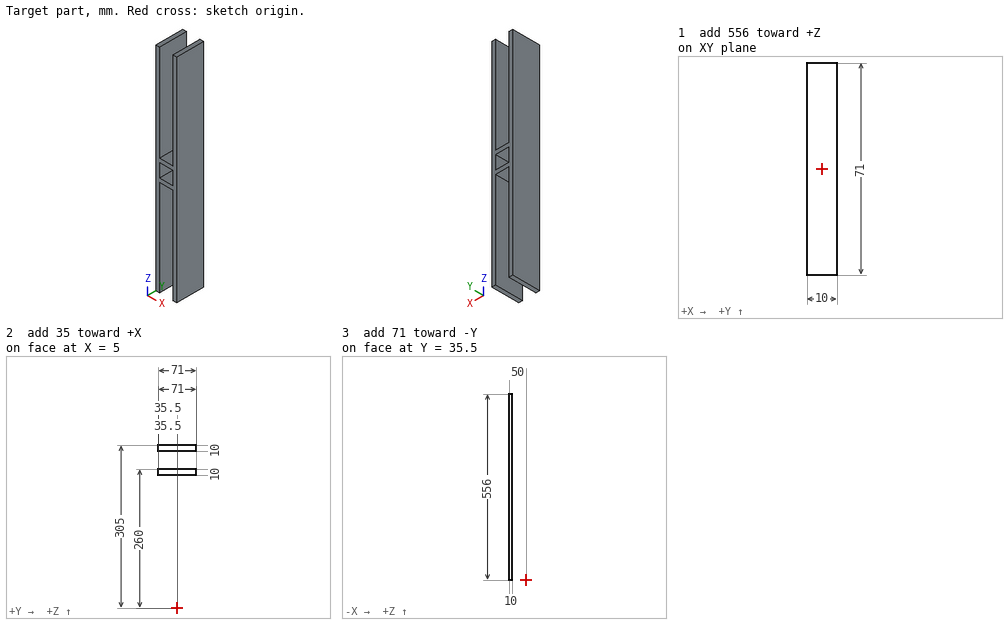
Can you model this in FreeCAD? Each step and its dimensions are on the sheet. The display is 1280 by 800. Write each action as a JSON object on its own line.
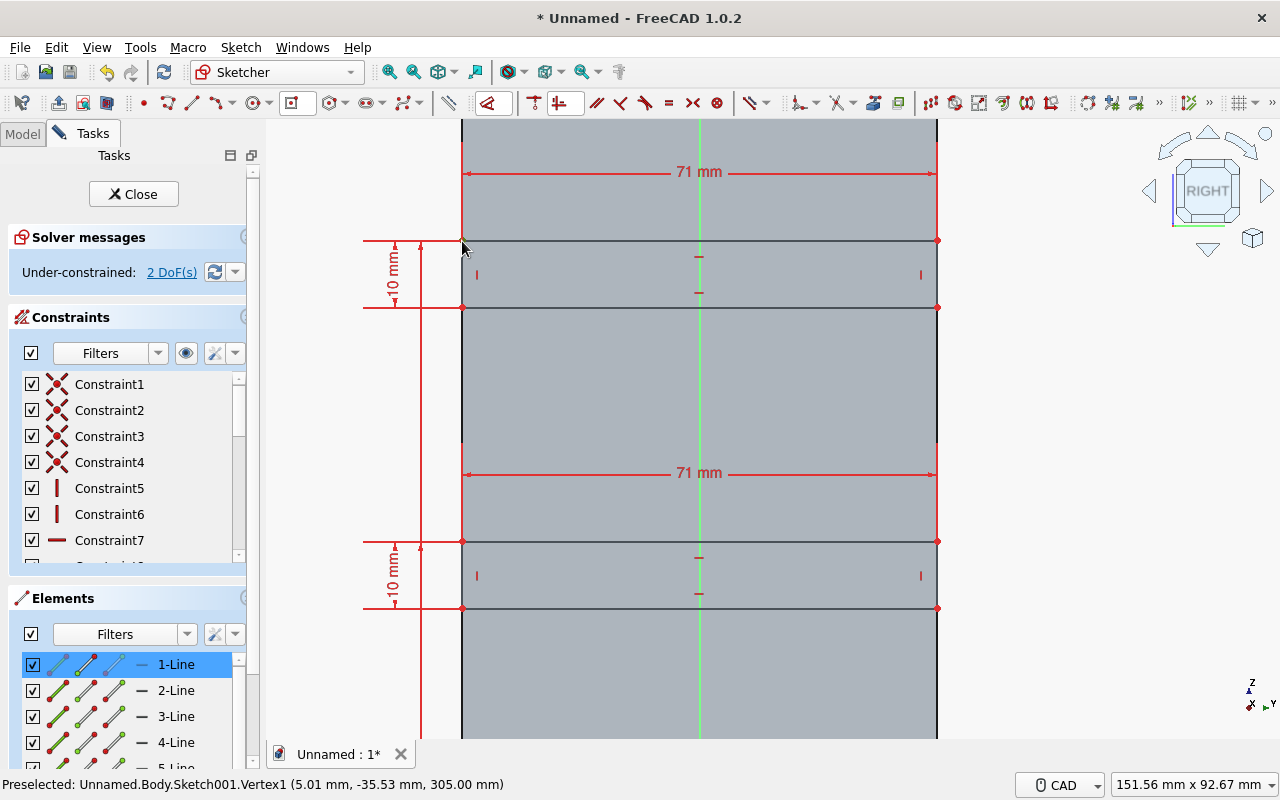
{"action": "key", "text": "l"}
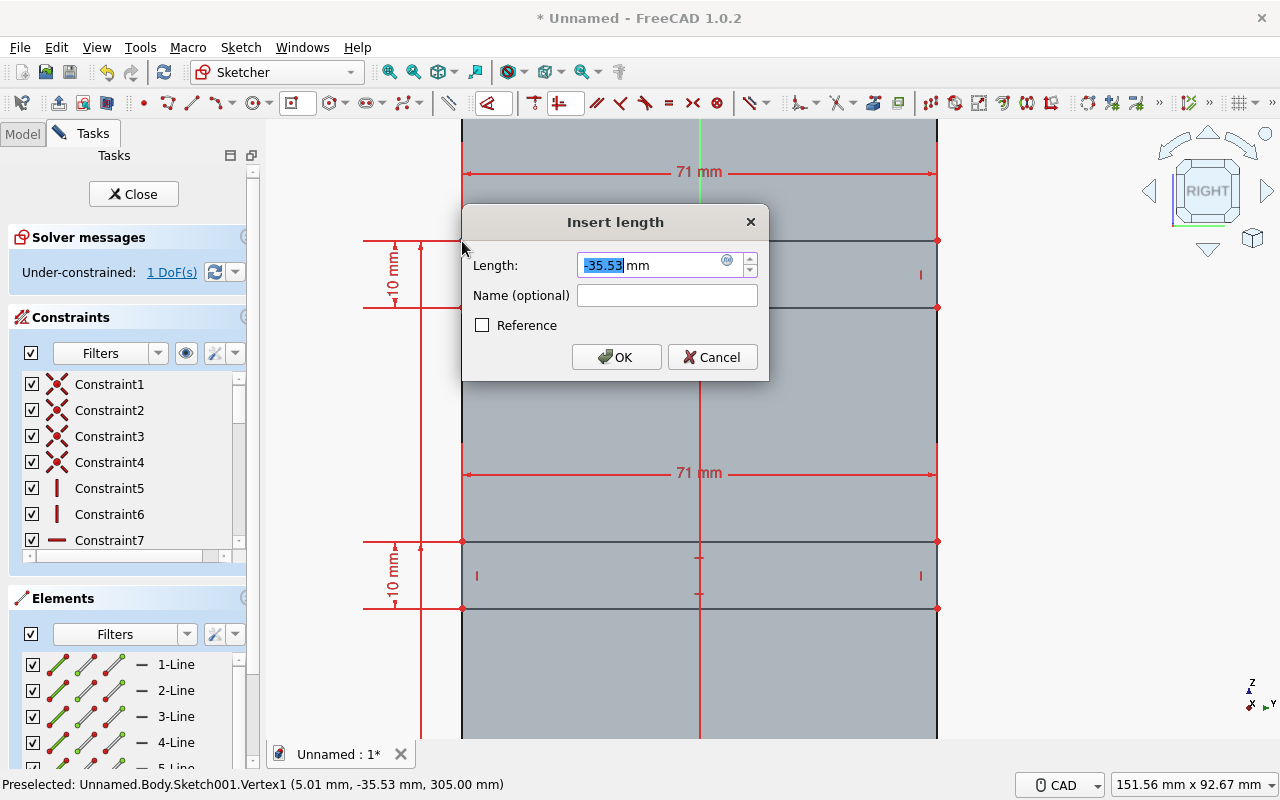
{"action": "type", "text": "-35.5"}
{"action": "key", "text": "Return"}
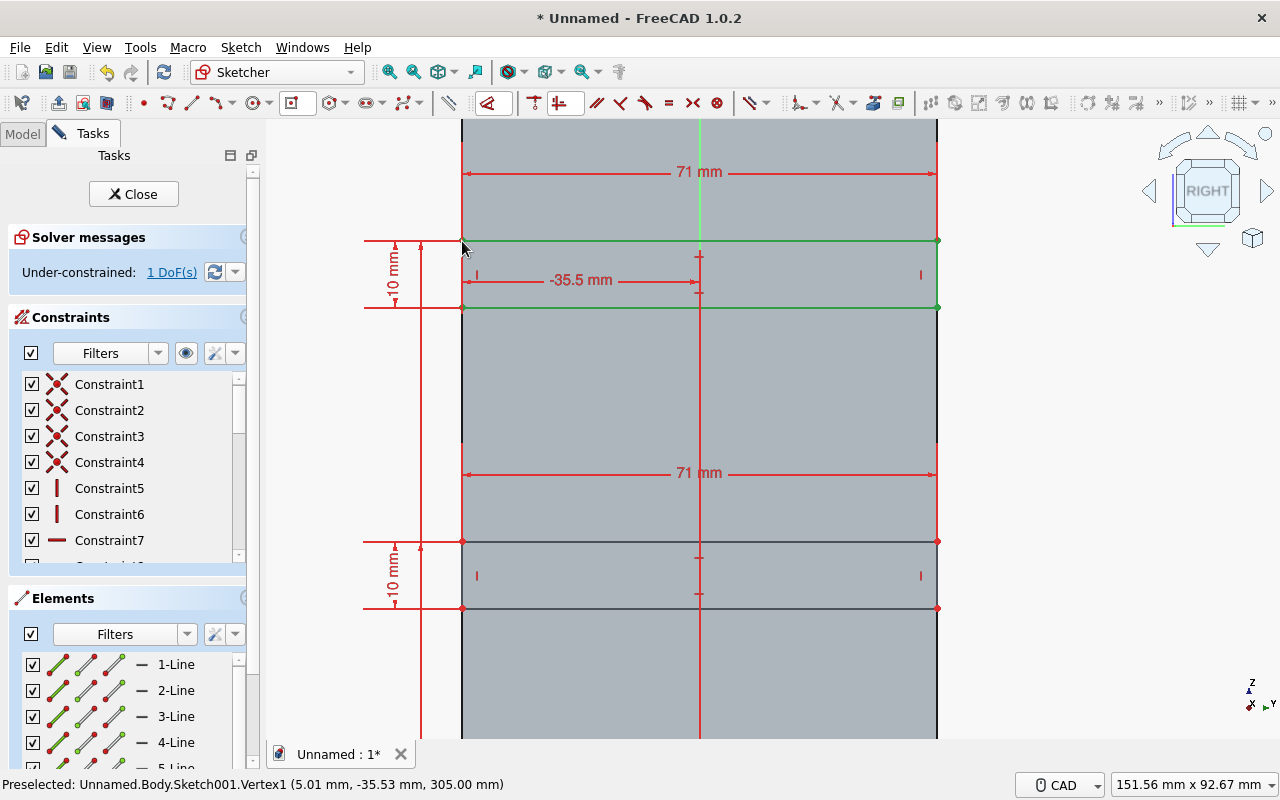
{"action": "left_click", "coordinate": [462, 542]}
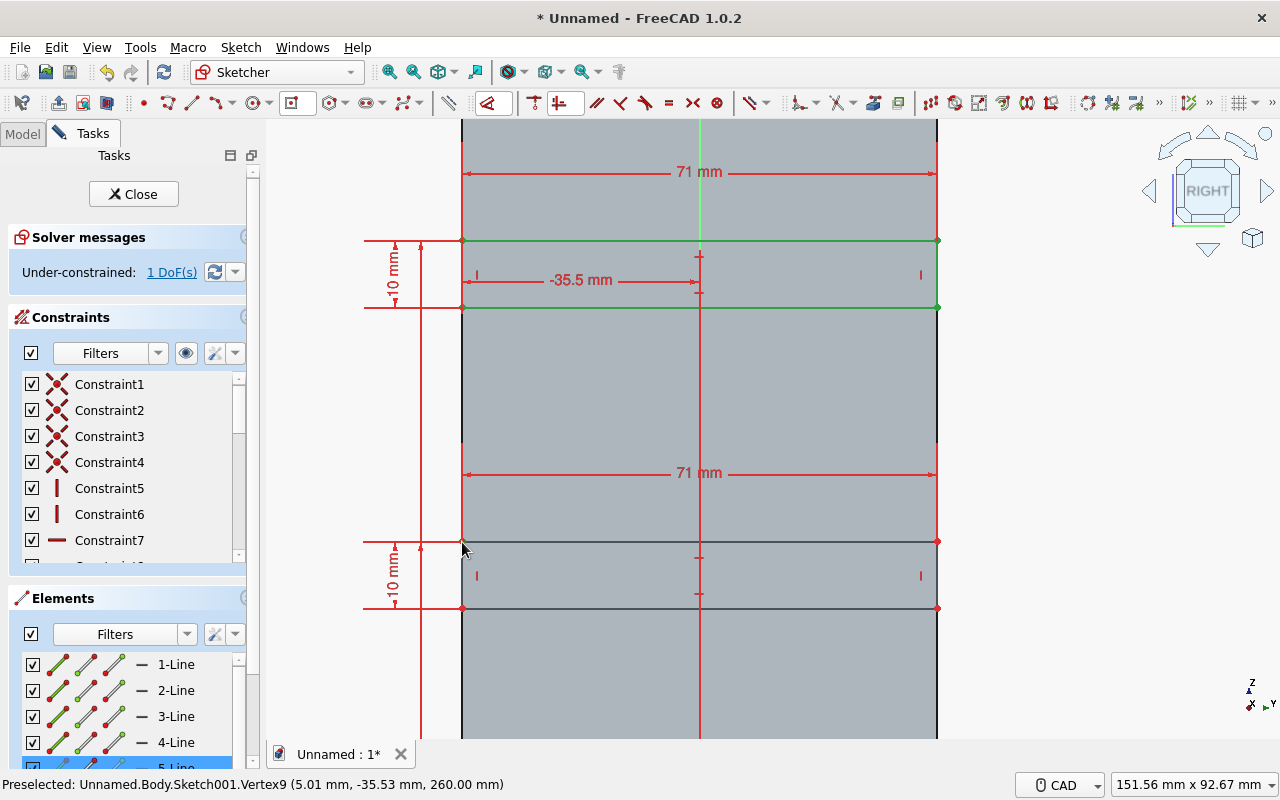
{"action": "left_click", "coordinate": [506, 104]}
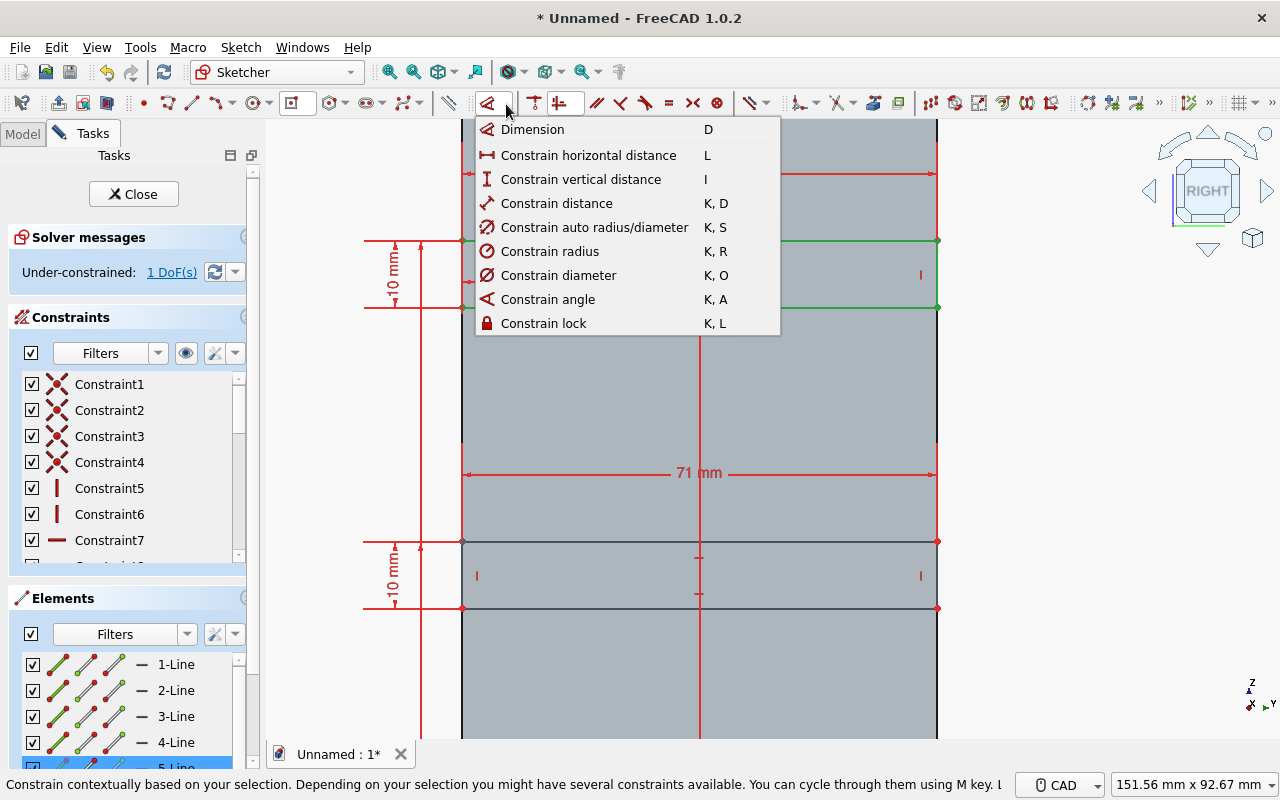
{"action": "left_click", "coordinate": [628, 155]}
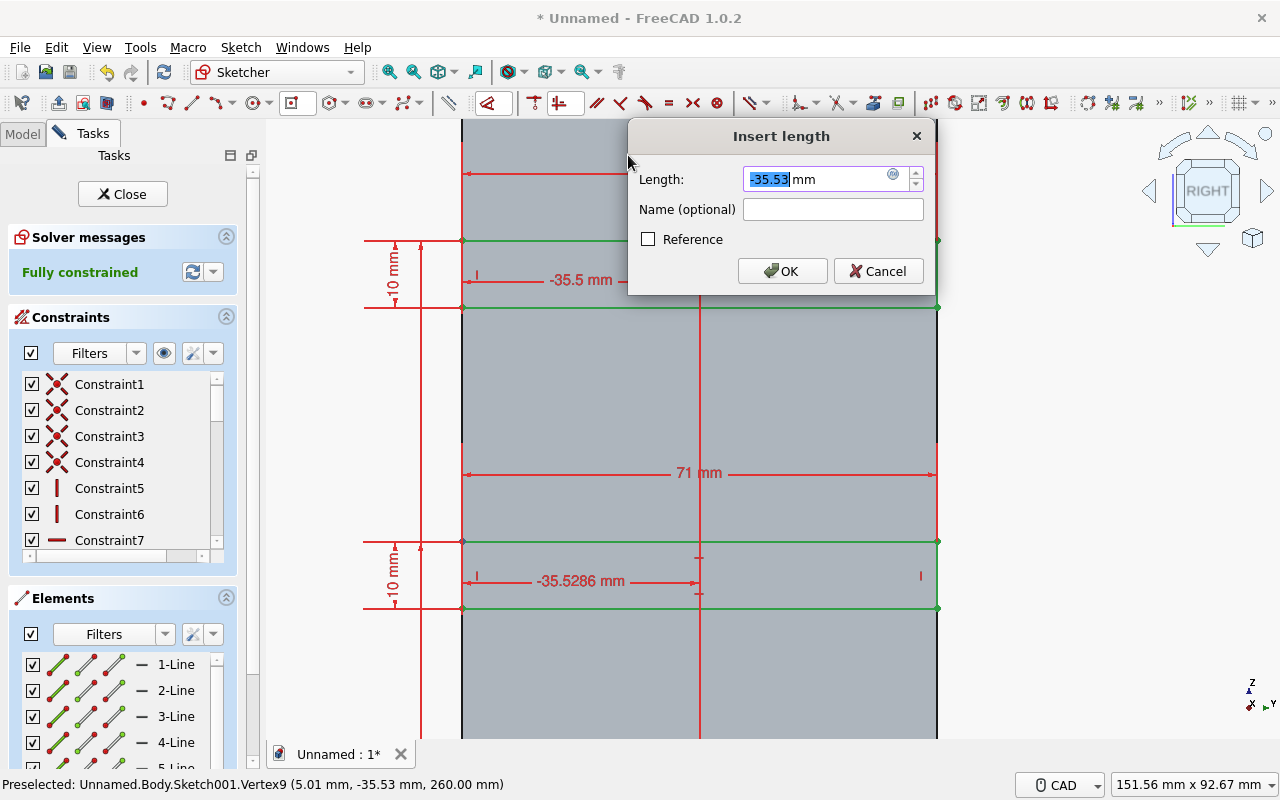
{"action": "type", "text": "-35.5"}
{"action": "key", "text": "Return"}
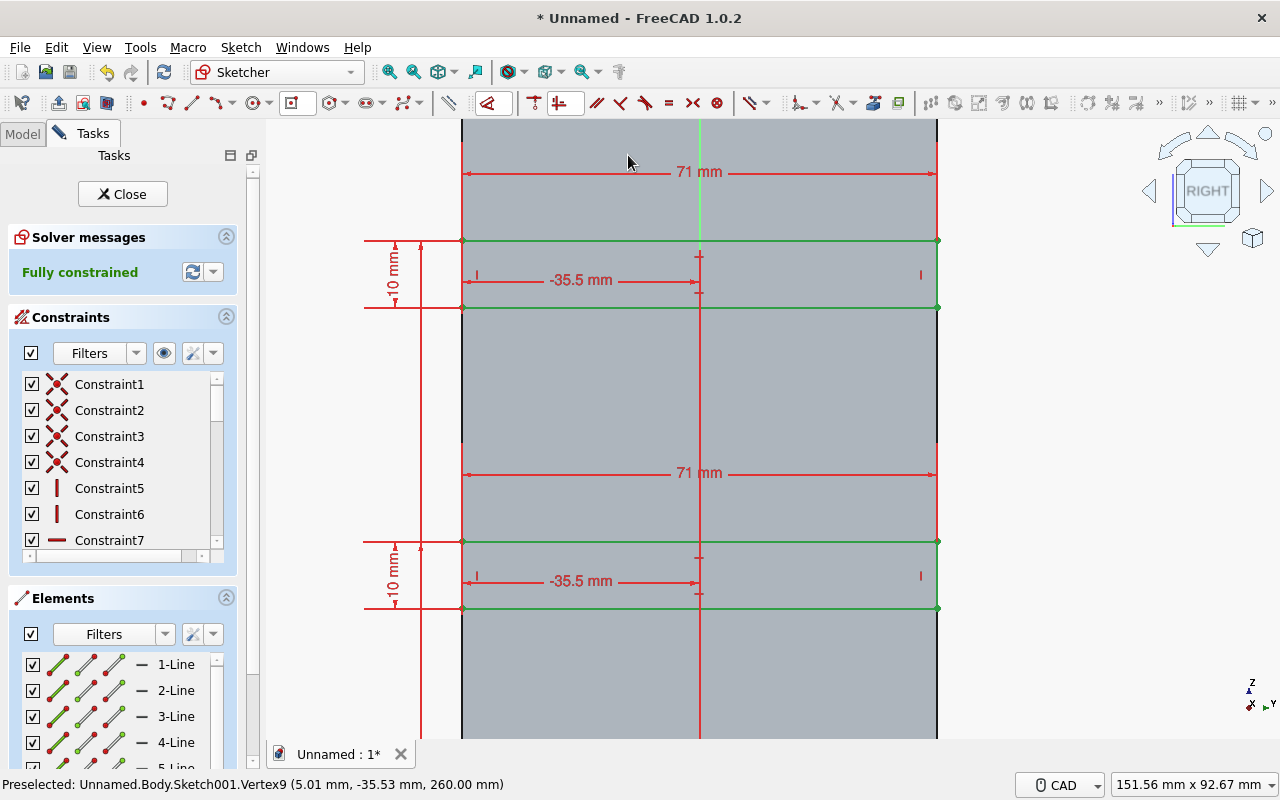
{"action": "left_click", "coordinate": [123, 194]}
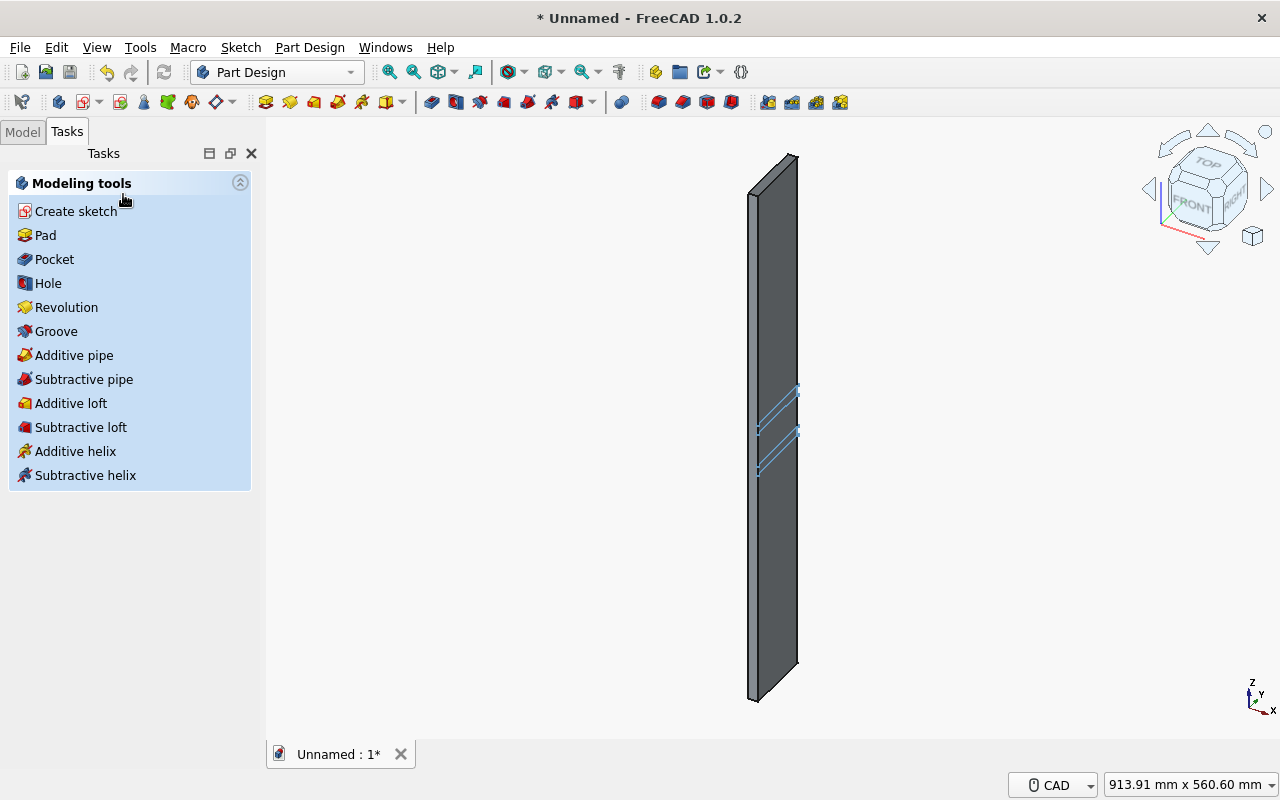
{"action": "left_click", "coordinate": [266, 102]}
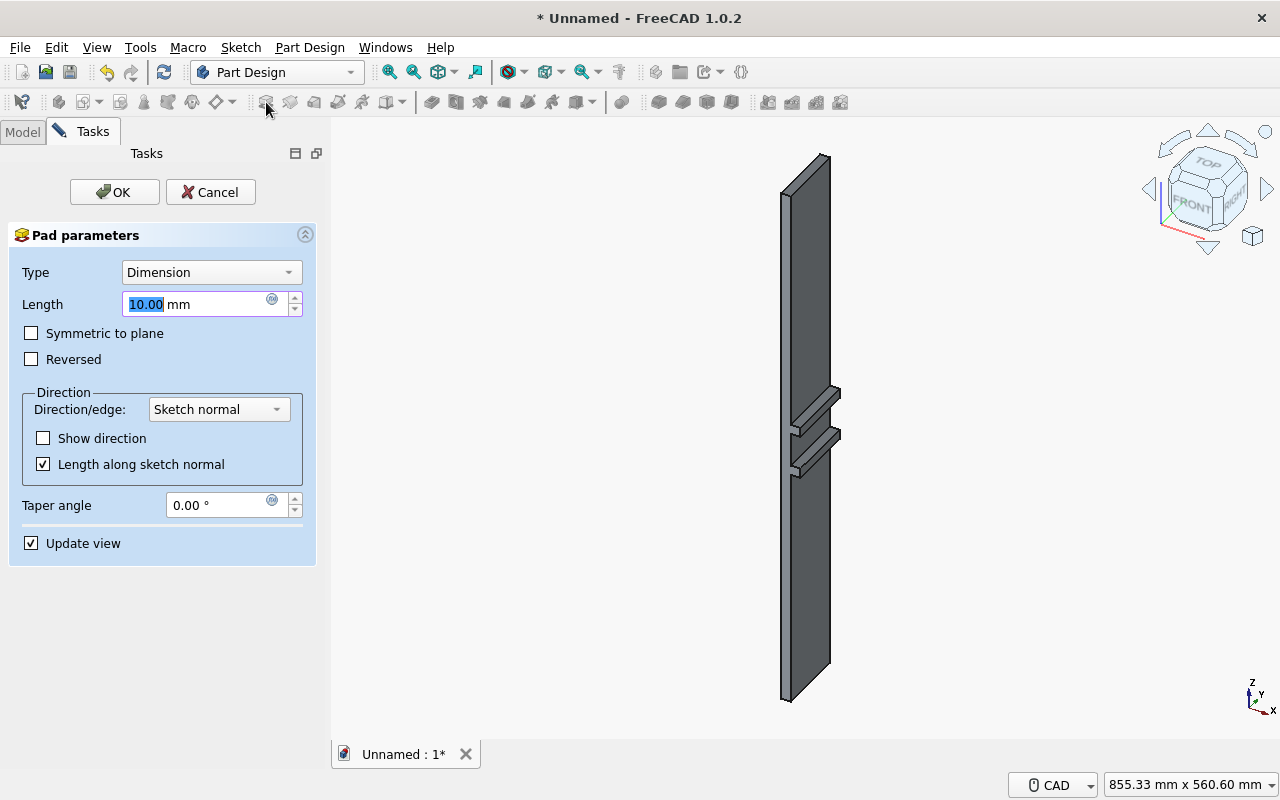
{"action": "type", "text": "35"}
{"action": "key", "text": "Tab"}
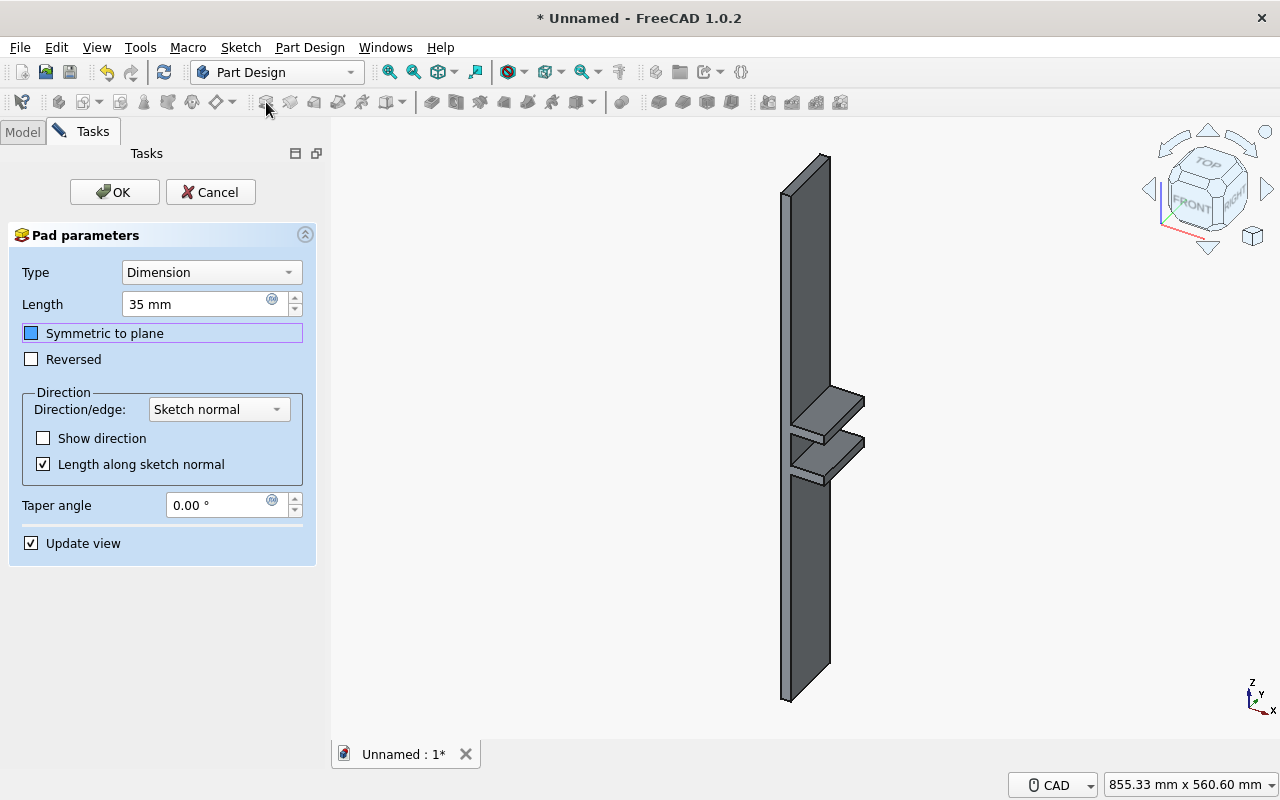
{"action": "left_click", "coordinate": [115, 192]}